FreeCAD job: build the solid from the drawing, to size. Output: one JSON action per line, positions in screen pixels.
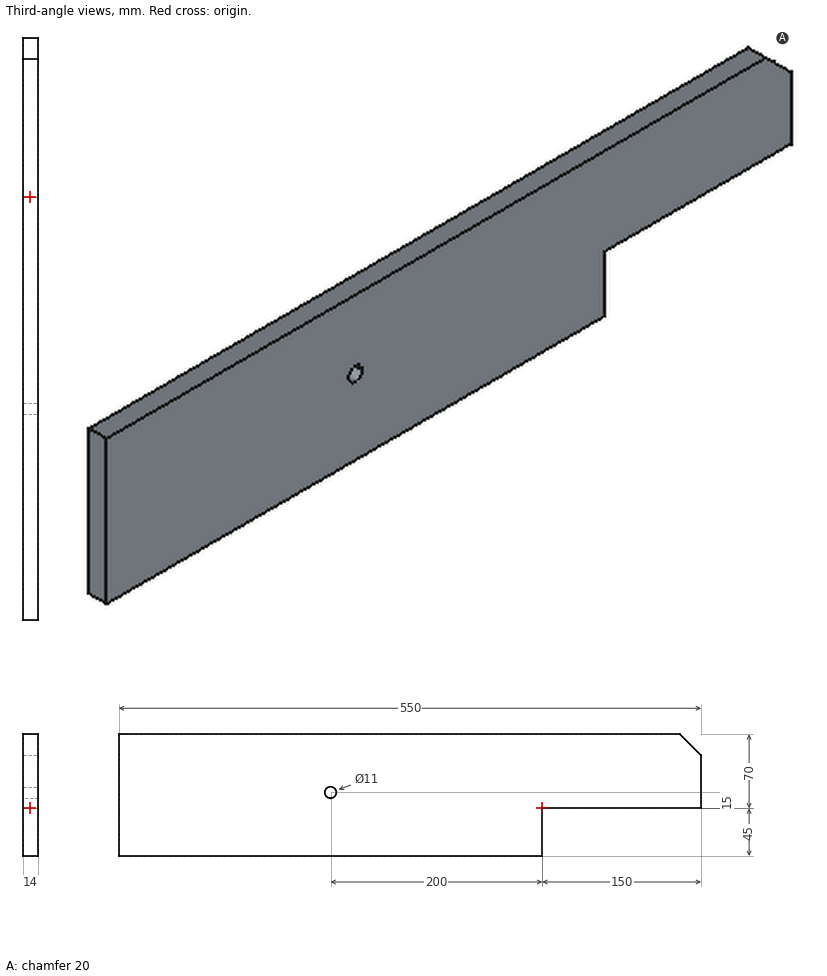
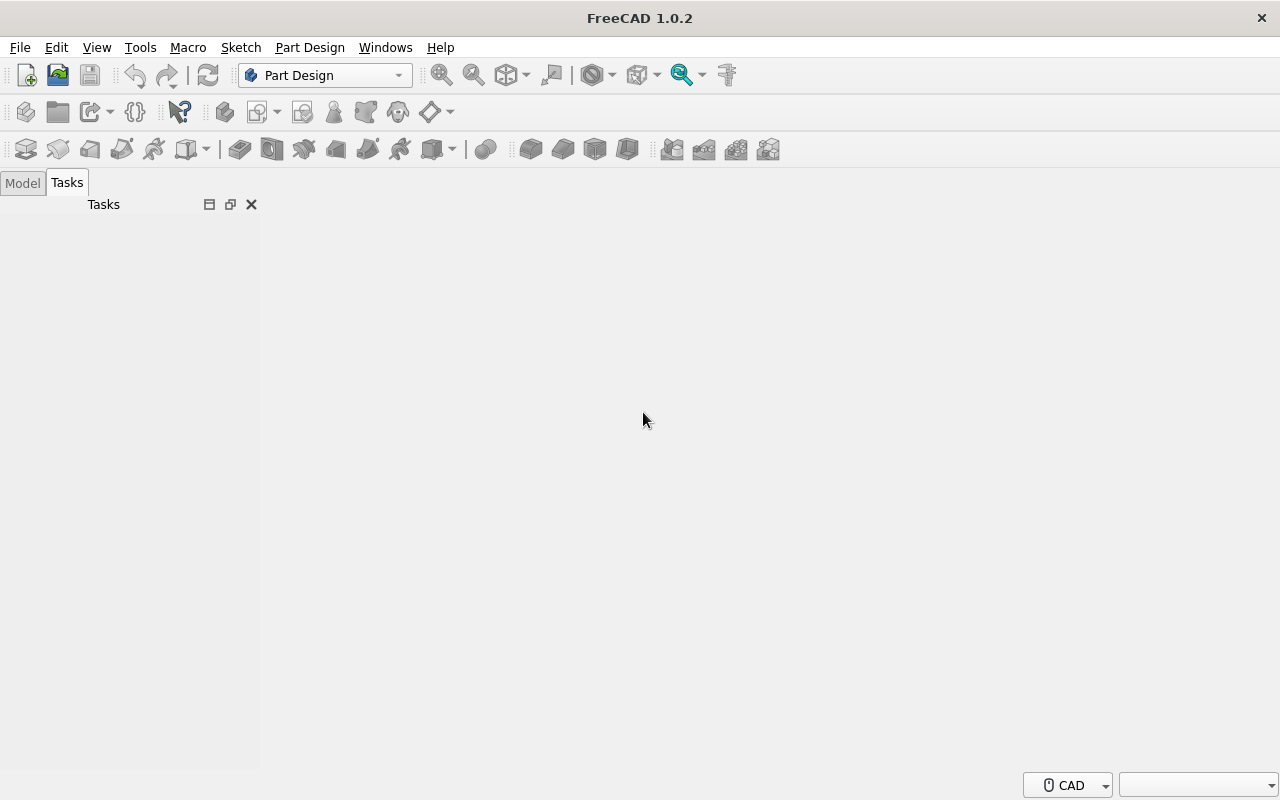
{"action": "left_click", "coordinate": [26, 76]}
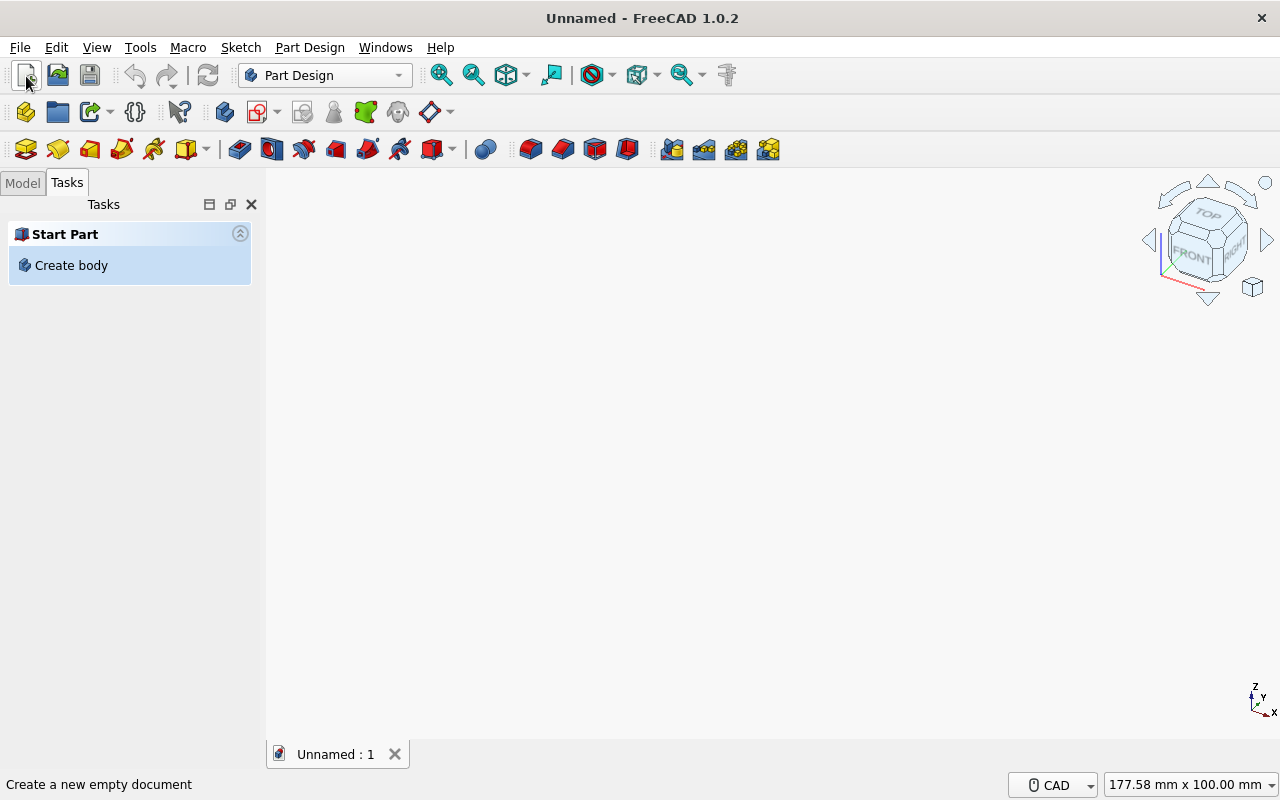
{"action": "left_click", "coordinate": [258, 112]}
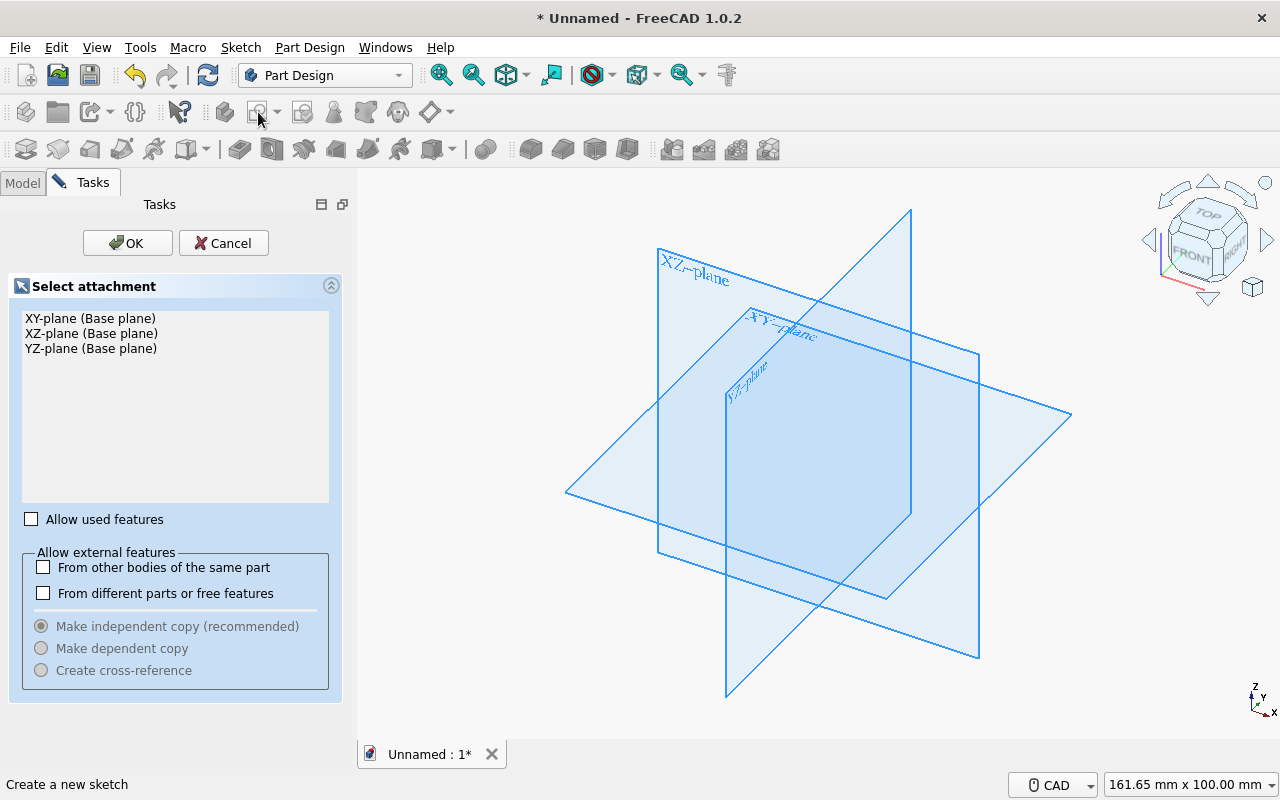
{"action": "left_click", "coordinate": [82, 348]}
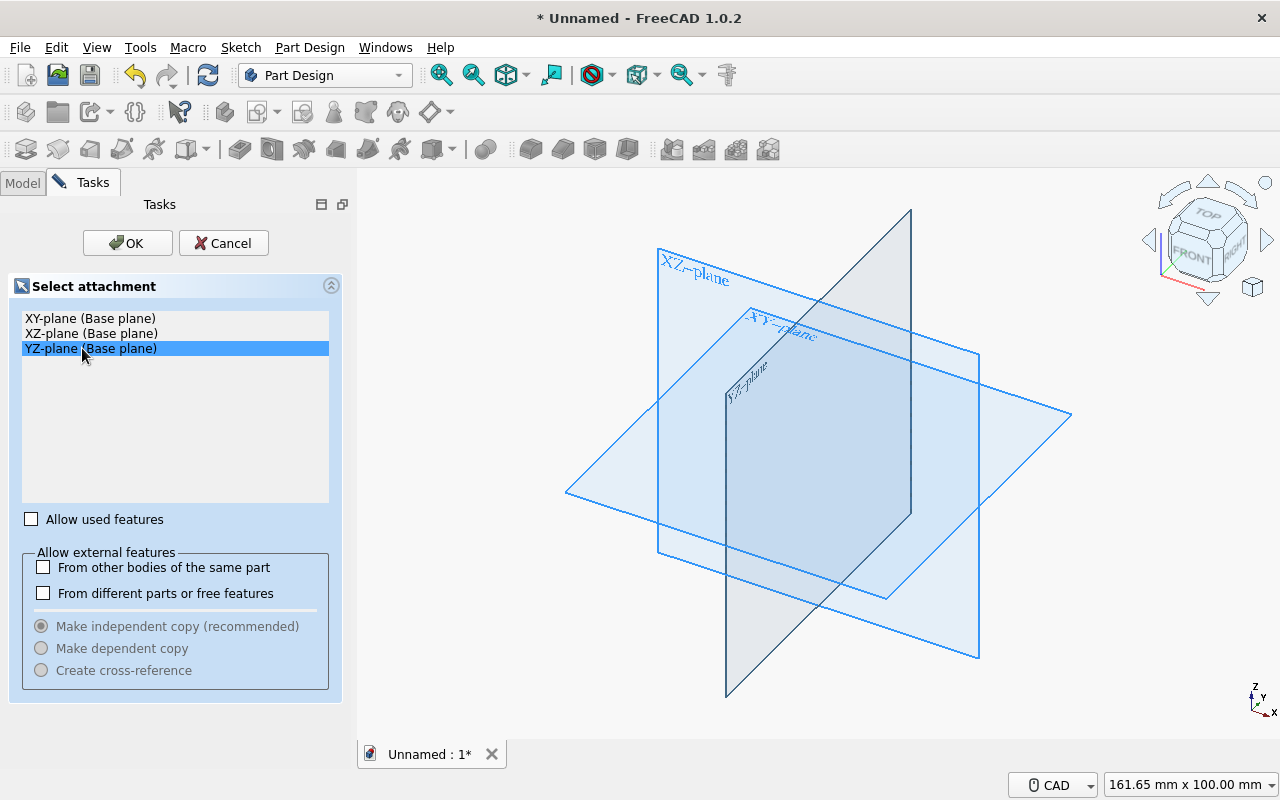
{"action": "left_click", "coordinate": [128, 243]}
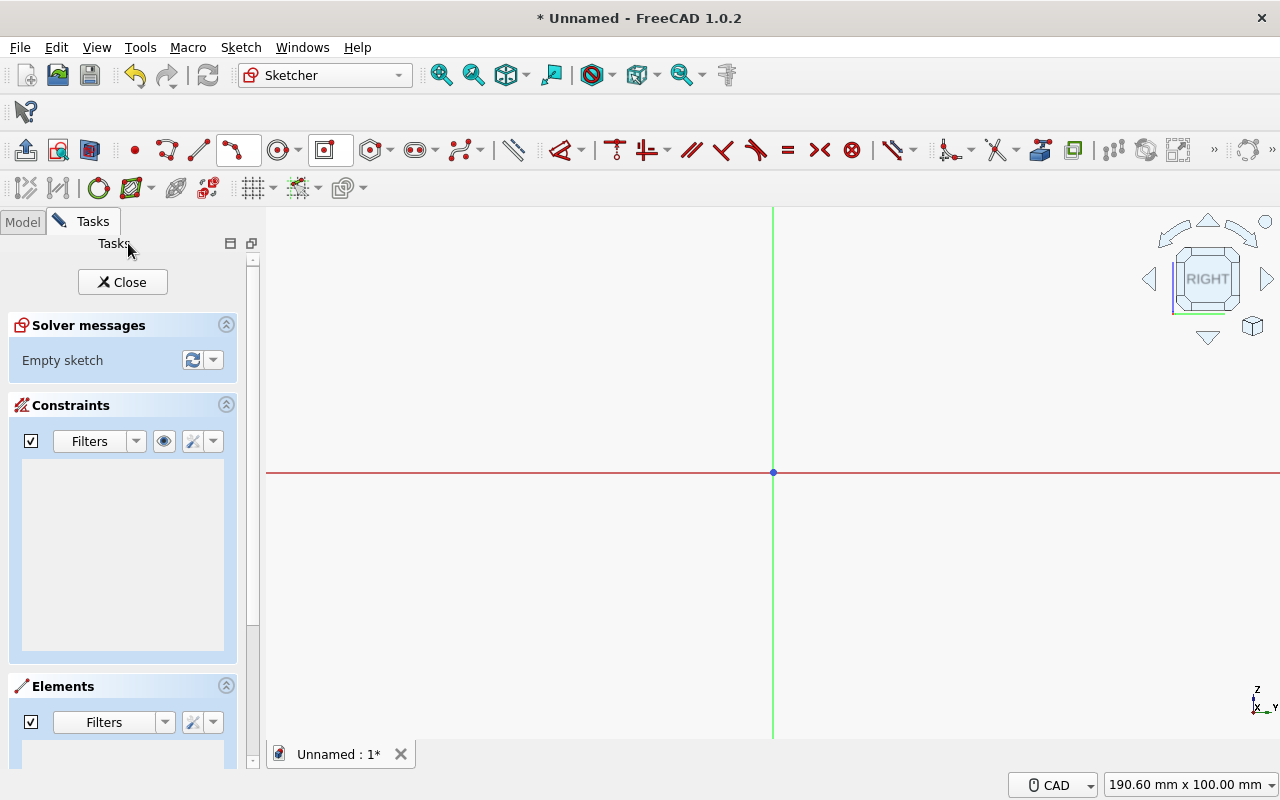
{"action": "scroll", "coordinate": [855, 490], "scroll_direction": "down", "scroll_amount": 8}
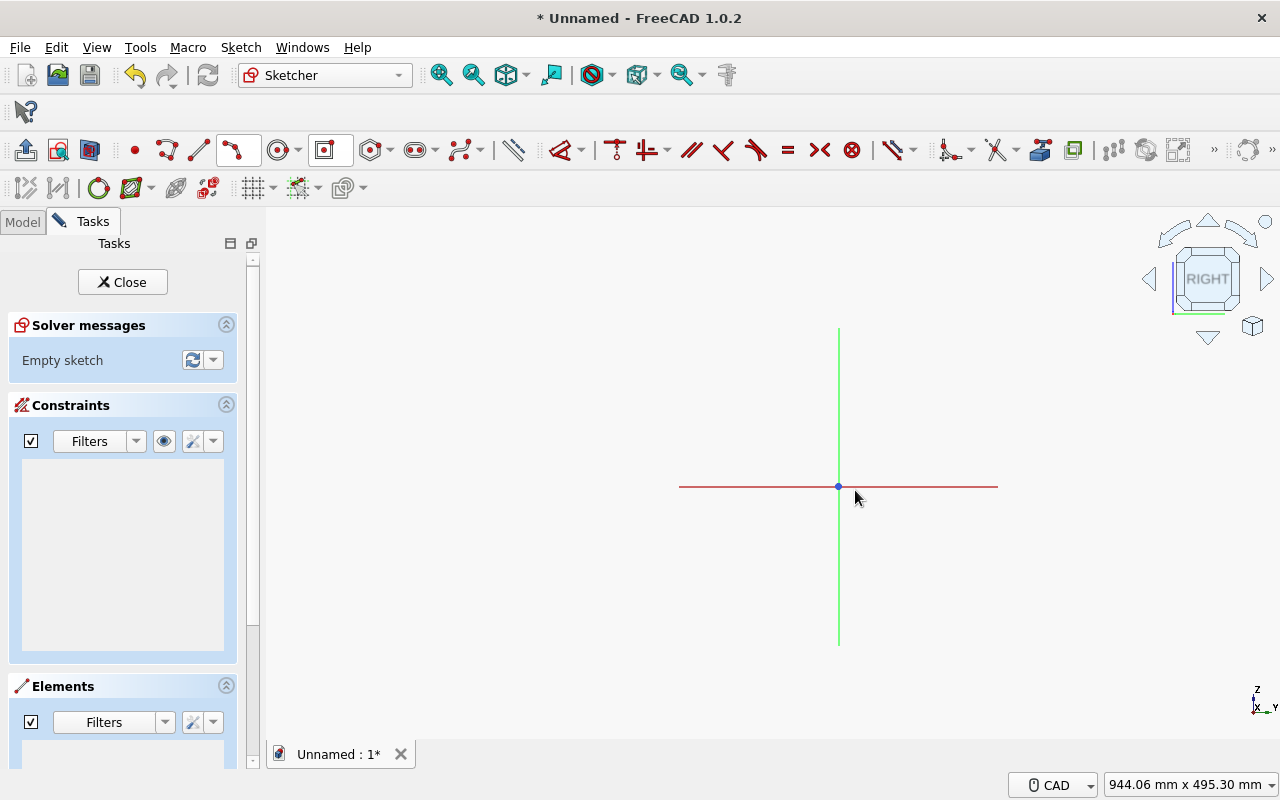
{"action": "left_click", "coordinate": [168, 150]}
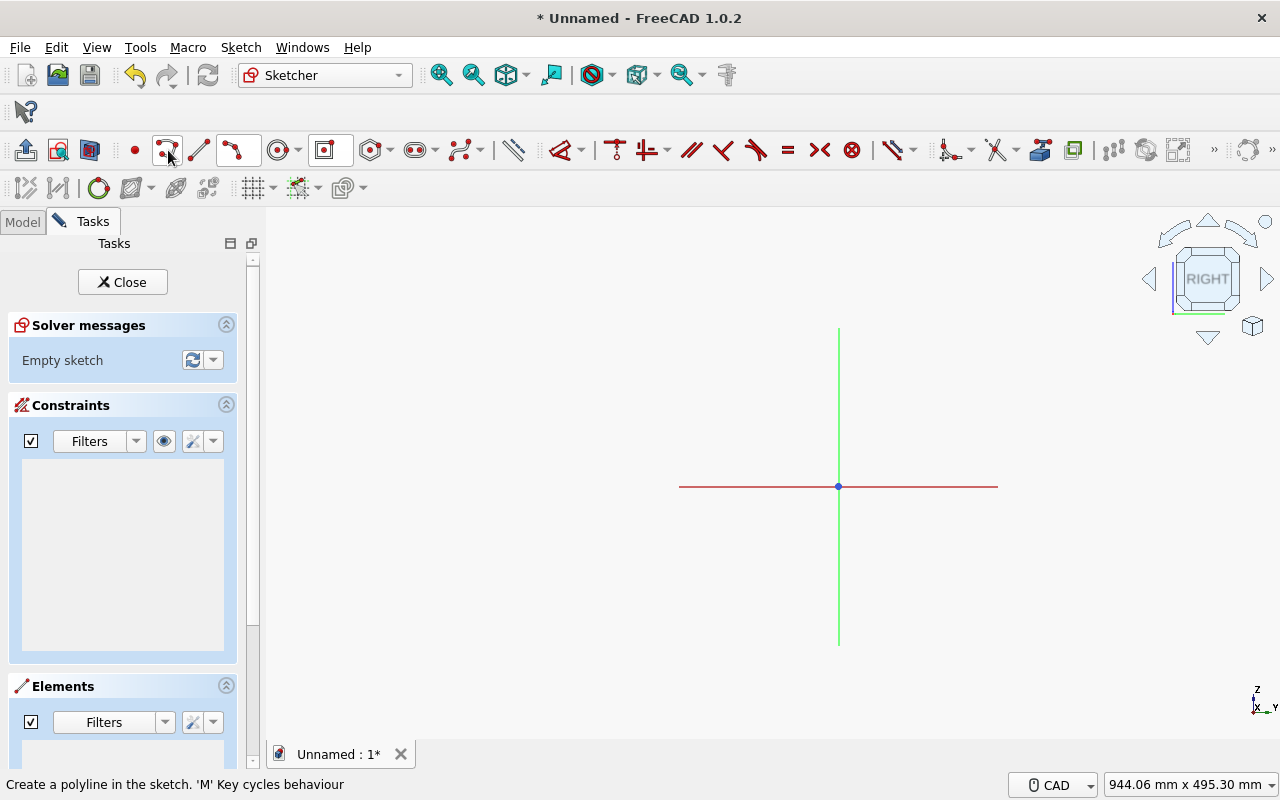
{"action": "left_click", "coordinate": [839, 487]}
{"action": "left_click", "coordinate": [1000, 478]}
{"action": "left_click", "coordinate": [1000, 412]}
{"action": "left_click", "coordinate": [409, 412]}
{"action": "left_click", "coordinate": [409, 535]}
{"action": "left_click", "coordinate": [830, 535]}
{"action": "left_click", "coordinate": [839, 487]}
{"action": "key", "text": "Escape"}
{"action": "key", "text": "Escape"}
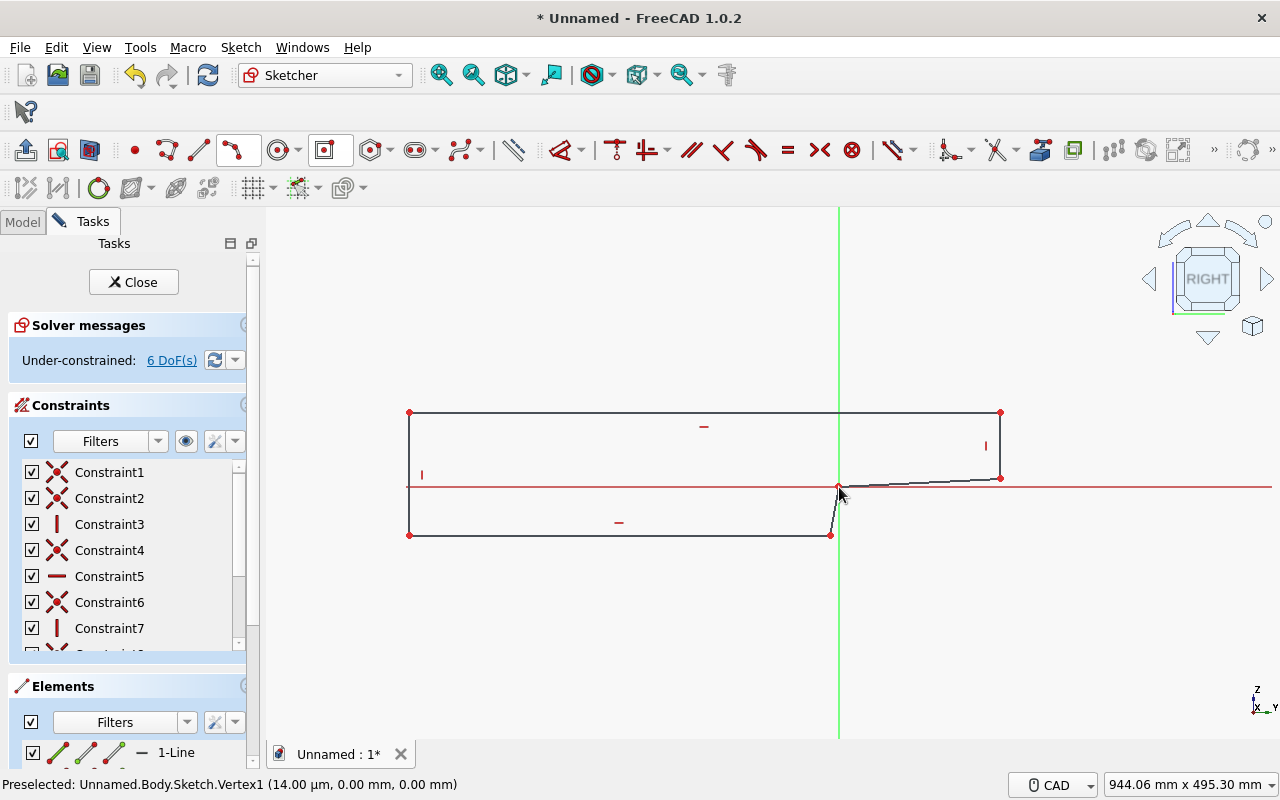
{"action": "left_click", "coordinate": [887, 485]}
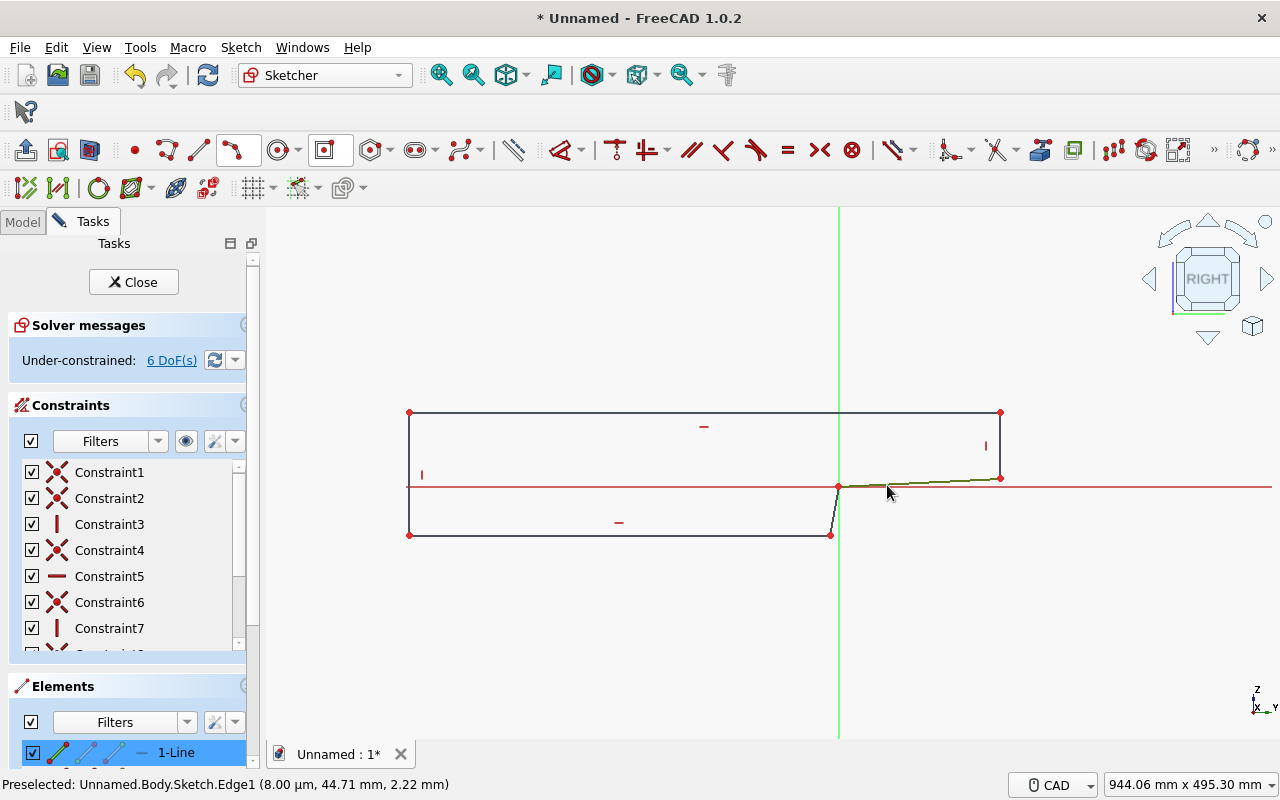
{"action": "left_click", "coordinate": [670, 150]}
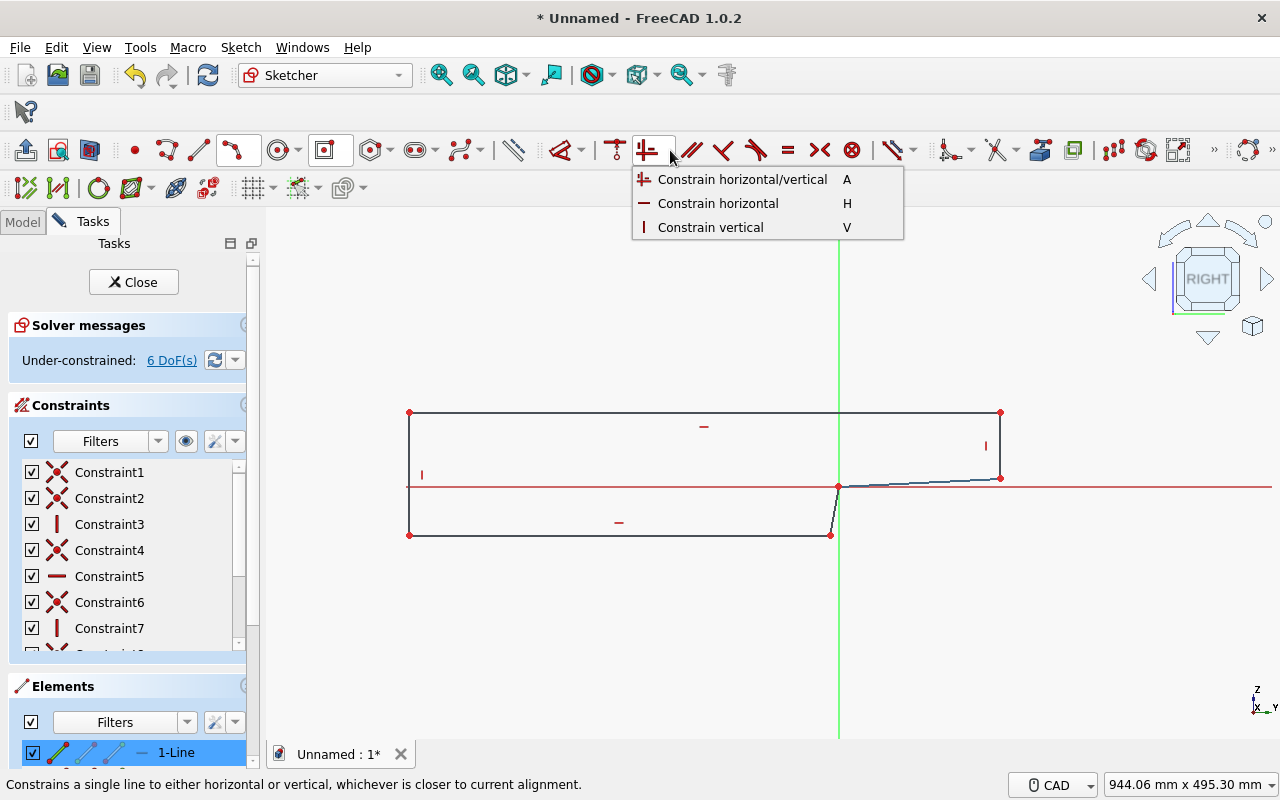
{"action": "left_click", "coordinate": [768, 203]}